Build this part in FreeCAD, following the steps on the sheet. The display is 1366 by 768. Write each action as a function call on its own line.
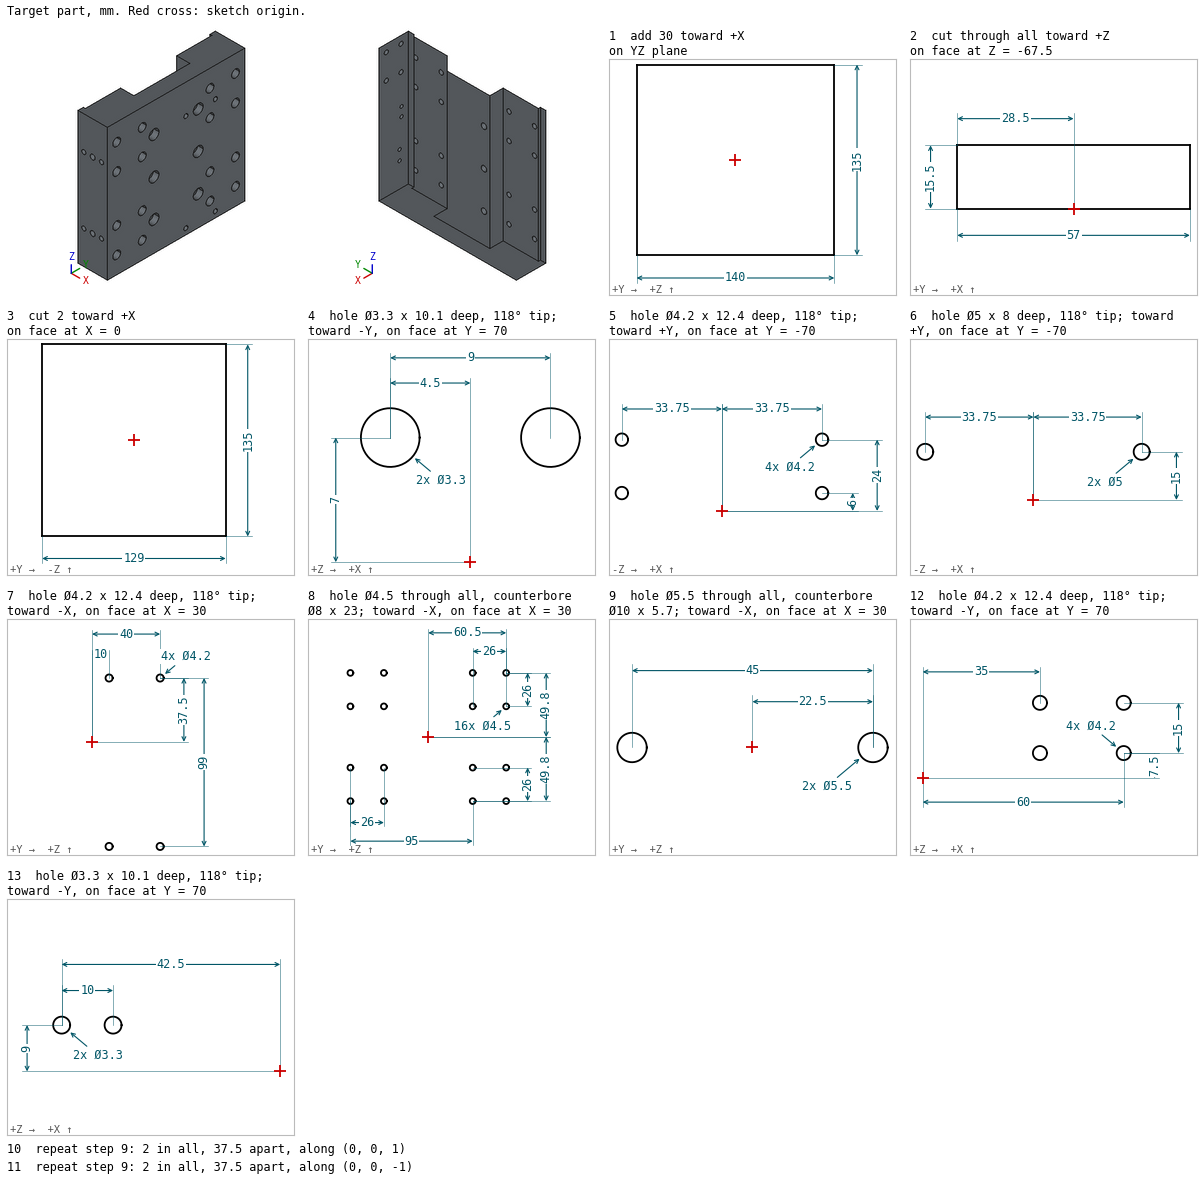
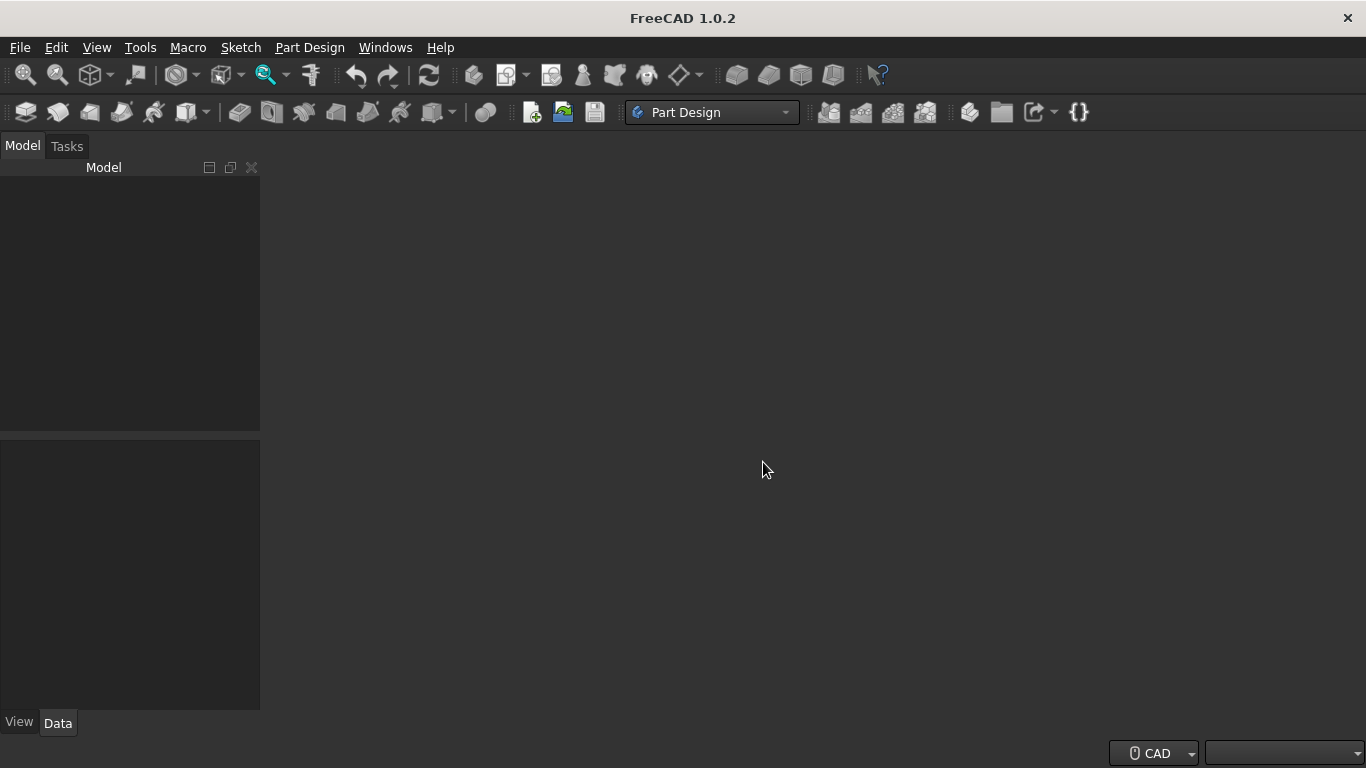
click(532, 112)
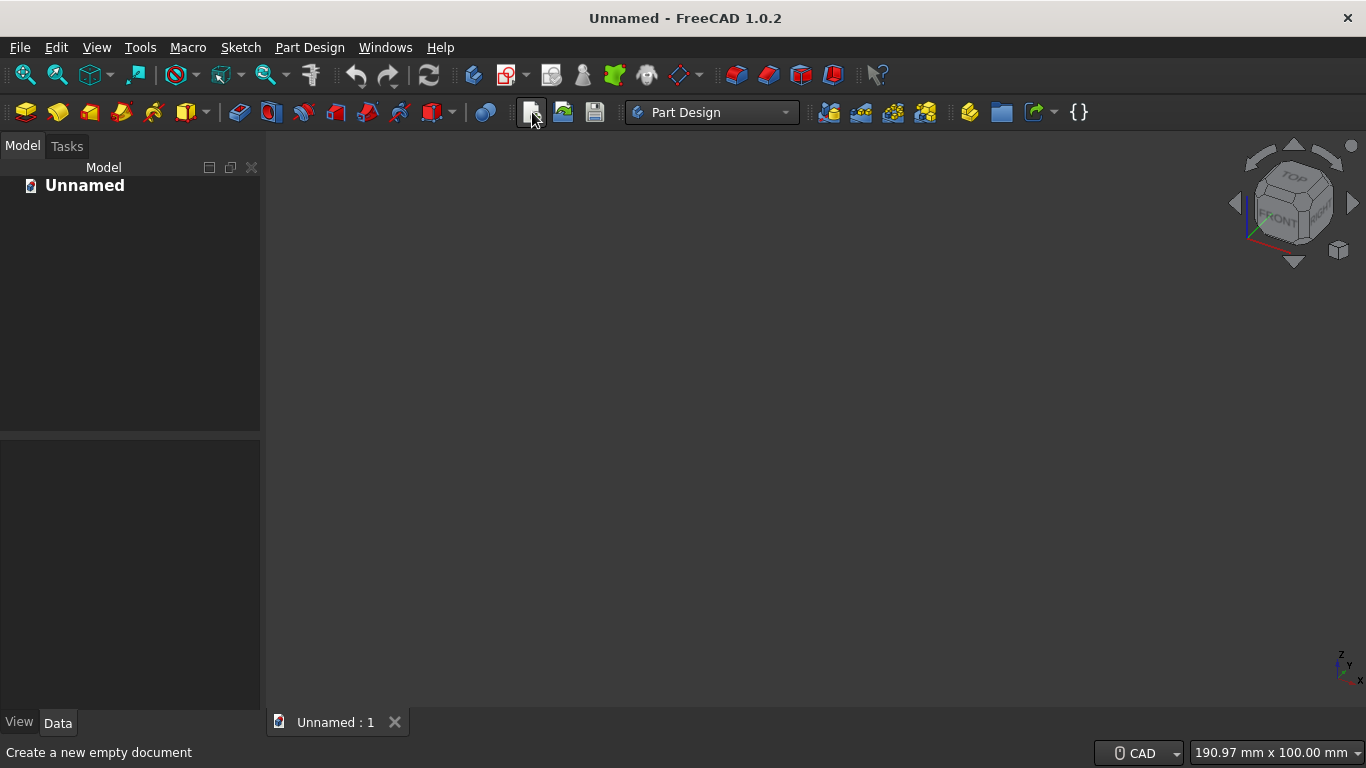
click(506, 76)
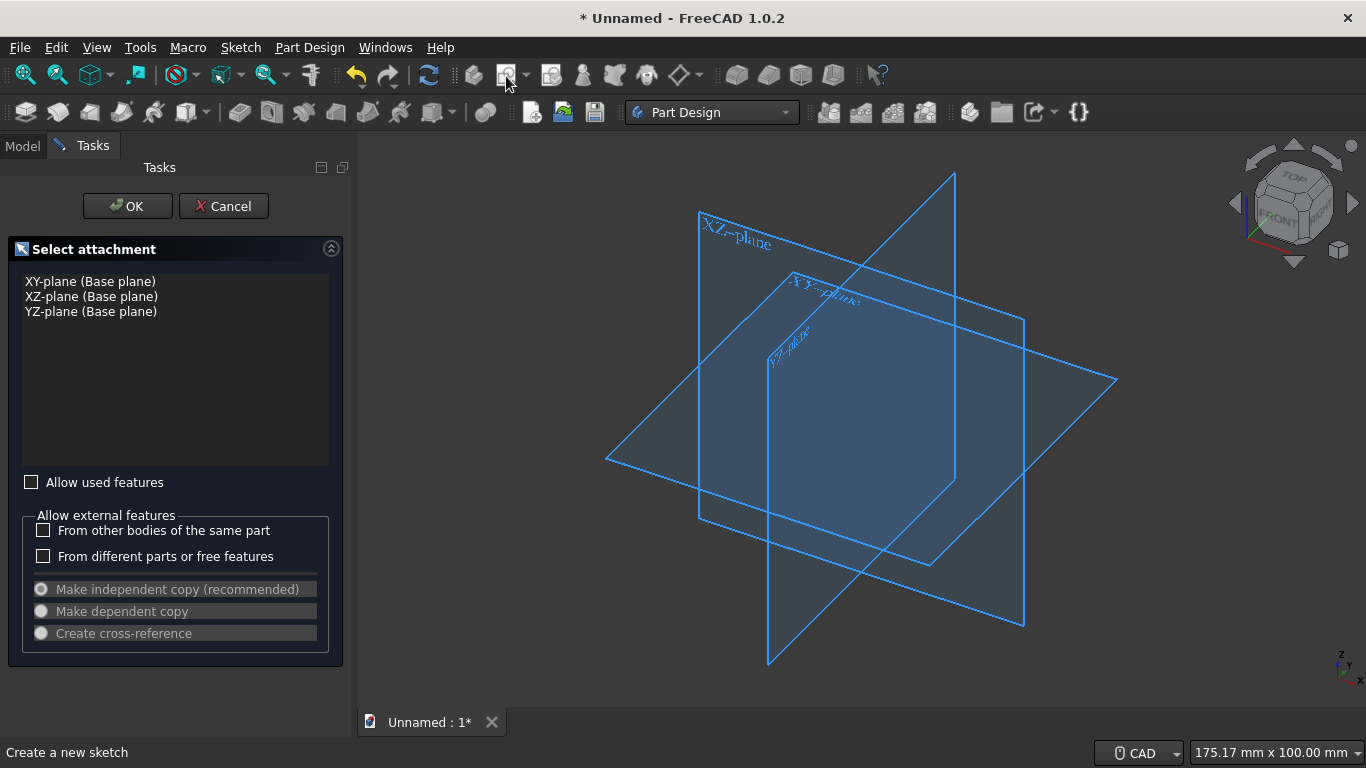
click(82, 312)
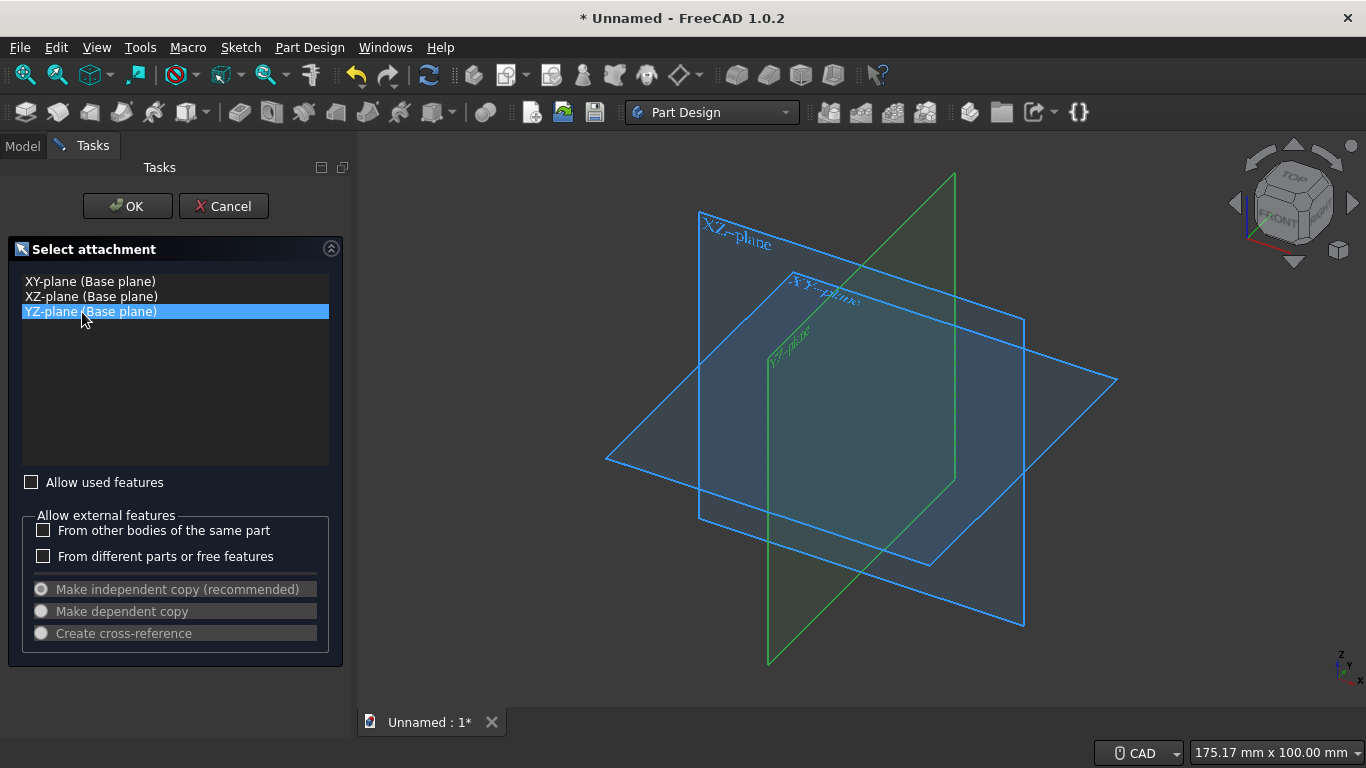
click(128, 206)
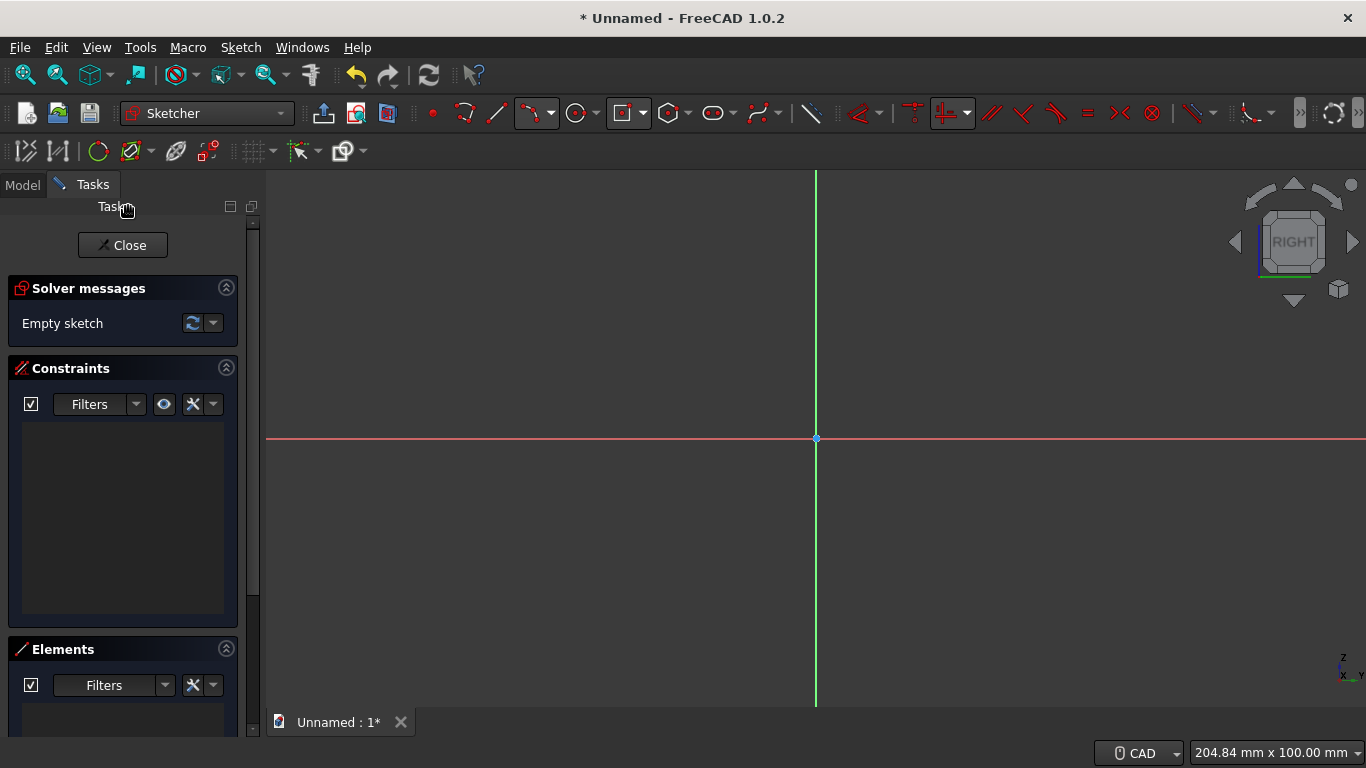
scroll(692, 438, down, 4)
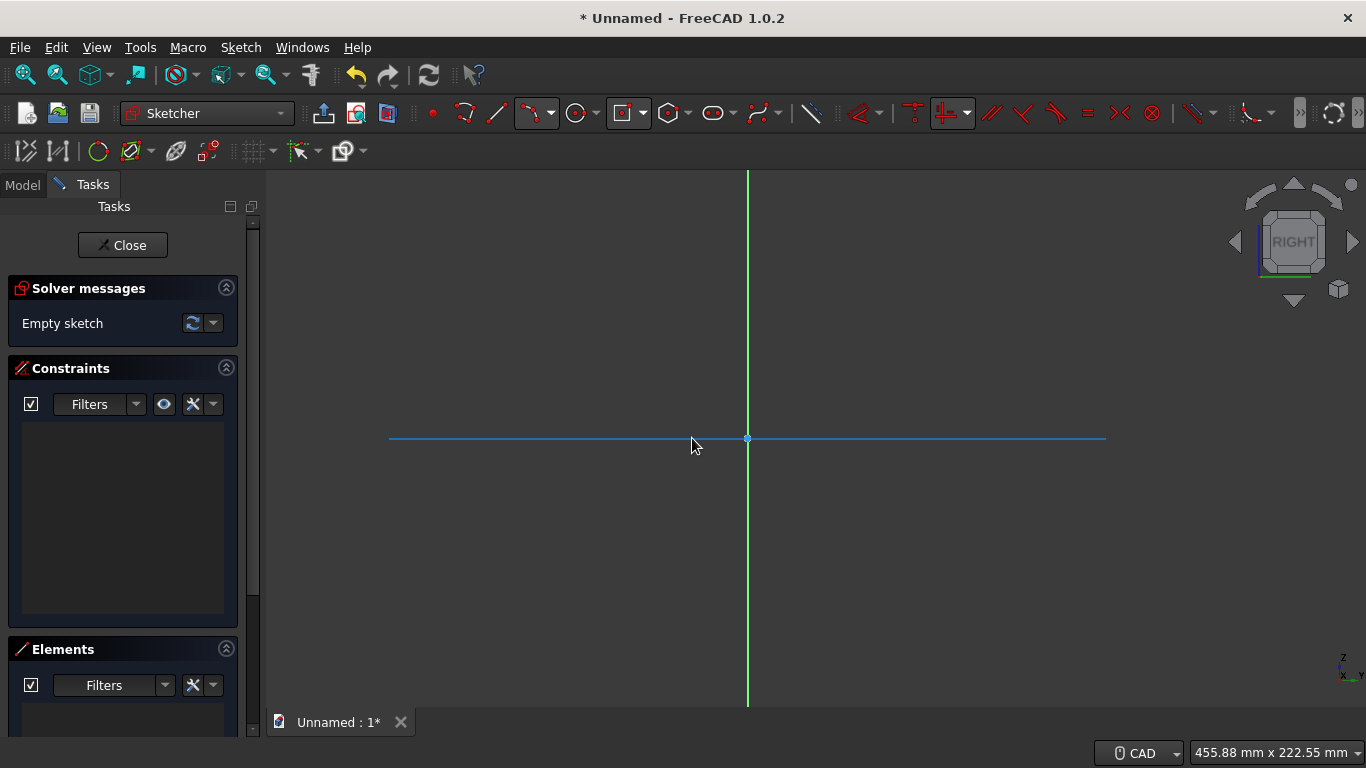
click(622, 114)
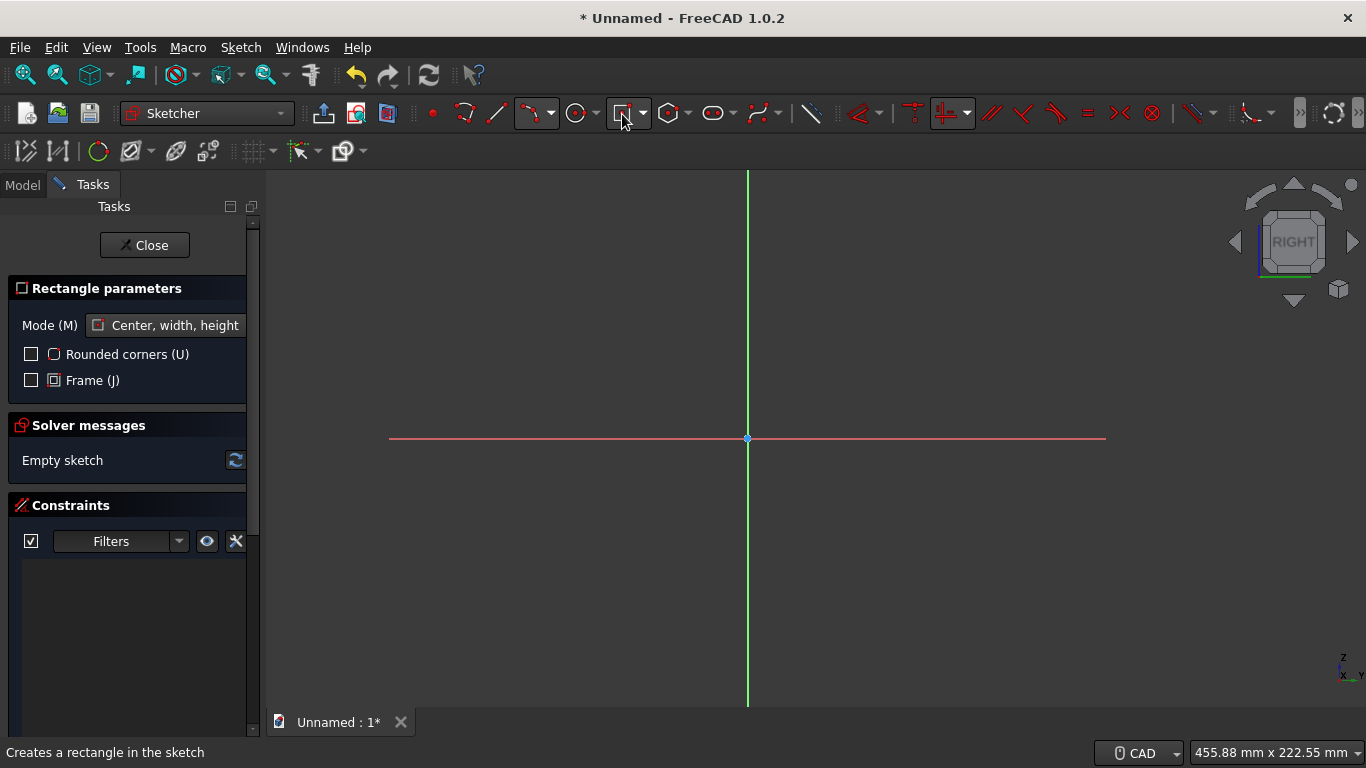
click(748, 438)
click(917, 276)
key(Escape)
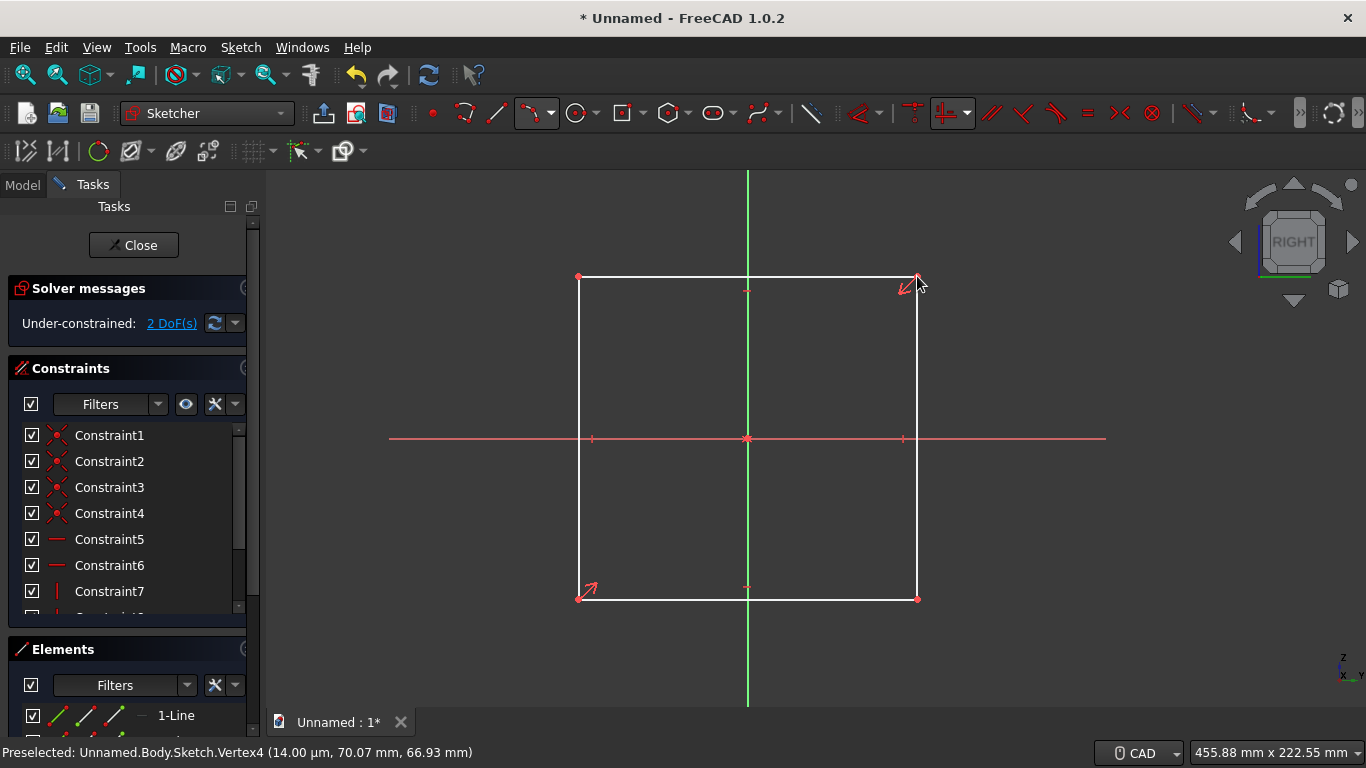
click(680, 600)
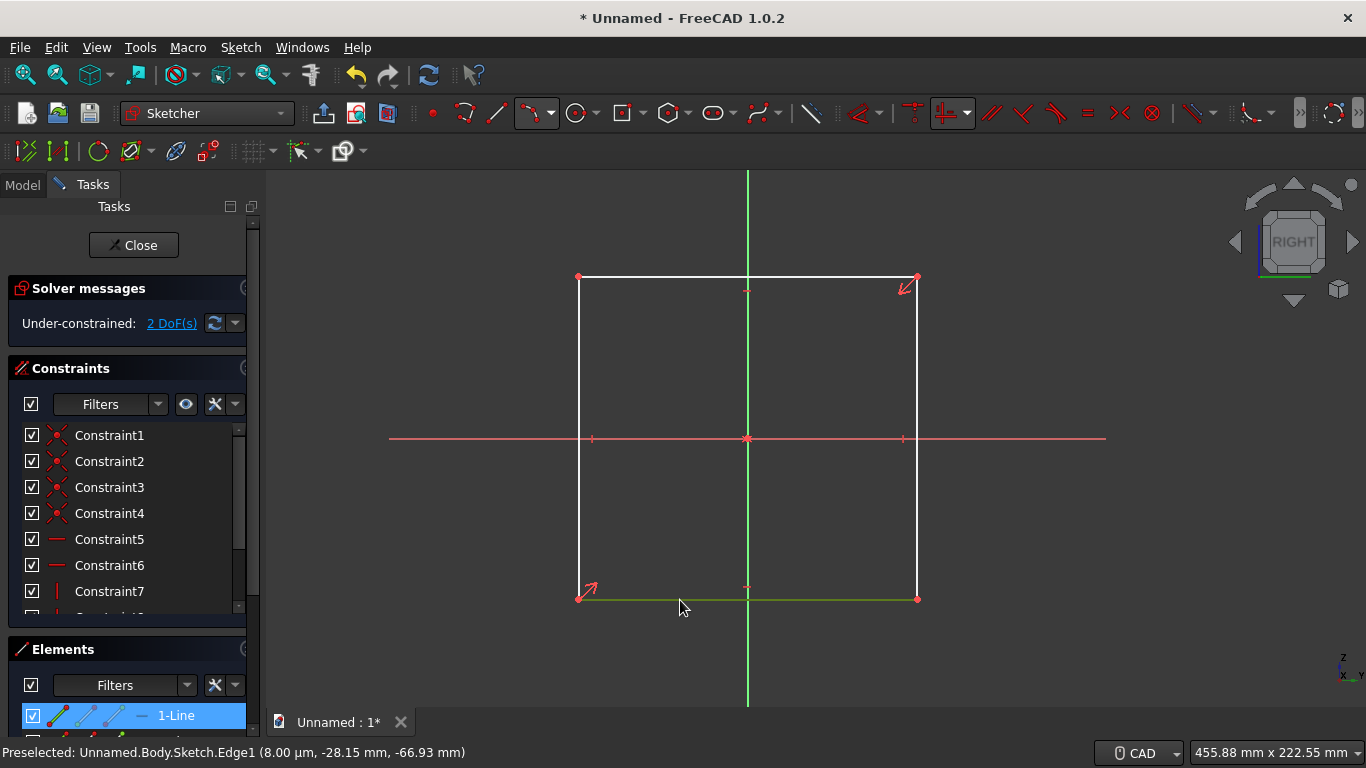
click(882, 114)